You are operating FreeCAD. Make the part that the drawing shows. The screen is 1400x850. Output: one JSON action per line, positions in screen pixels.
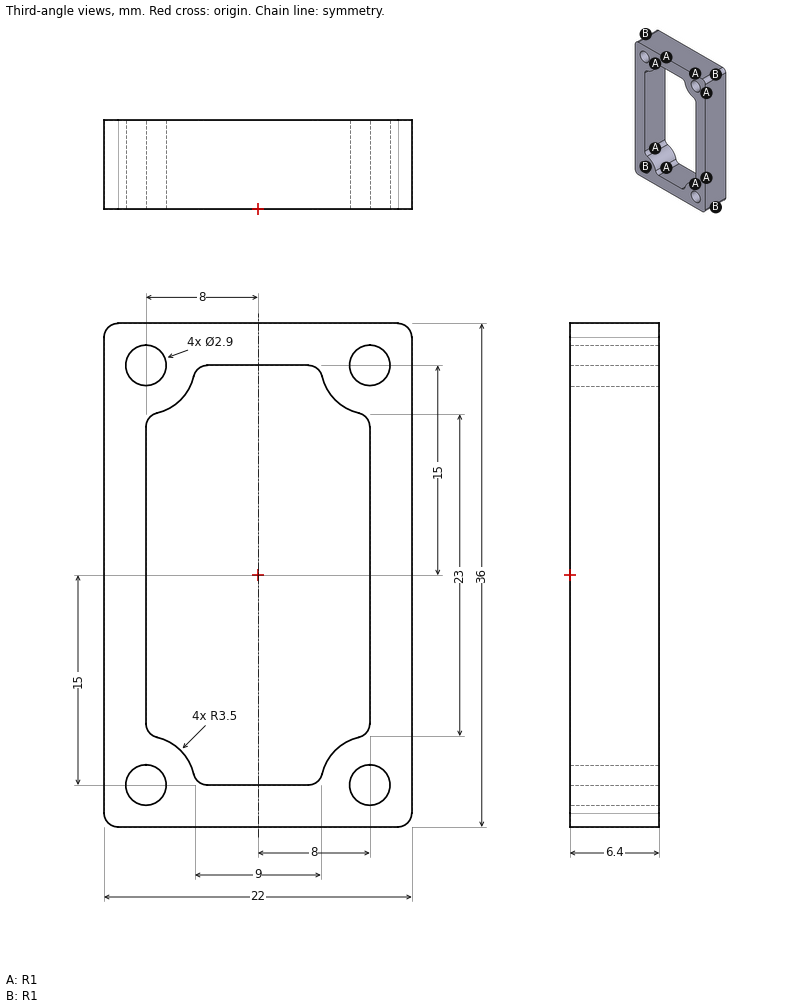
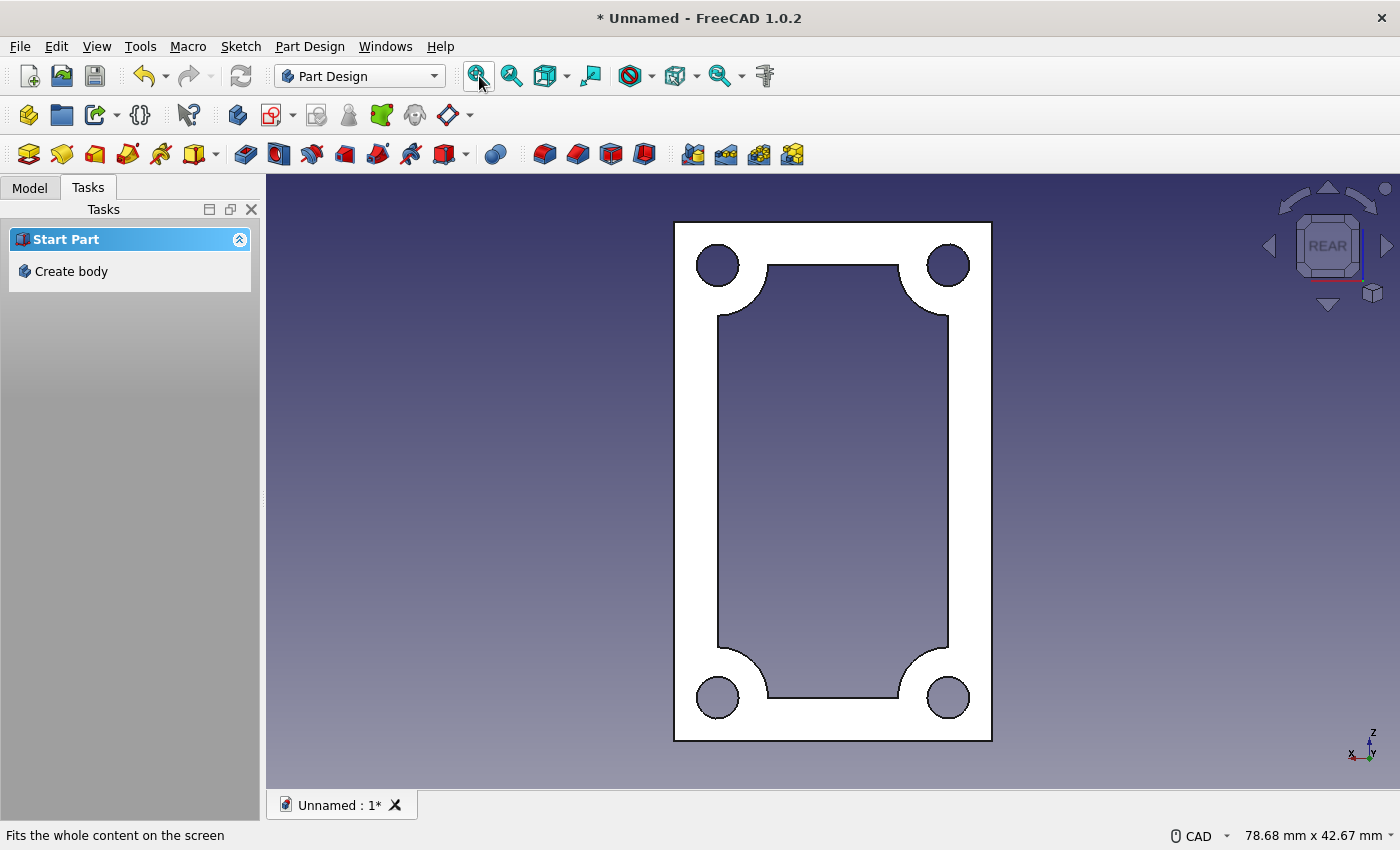
{"action": "key", "text": "6"}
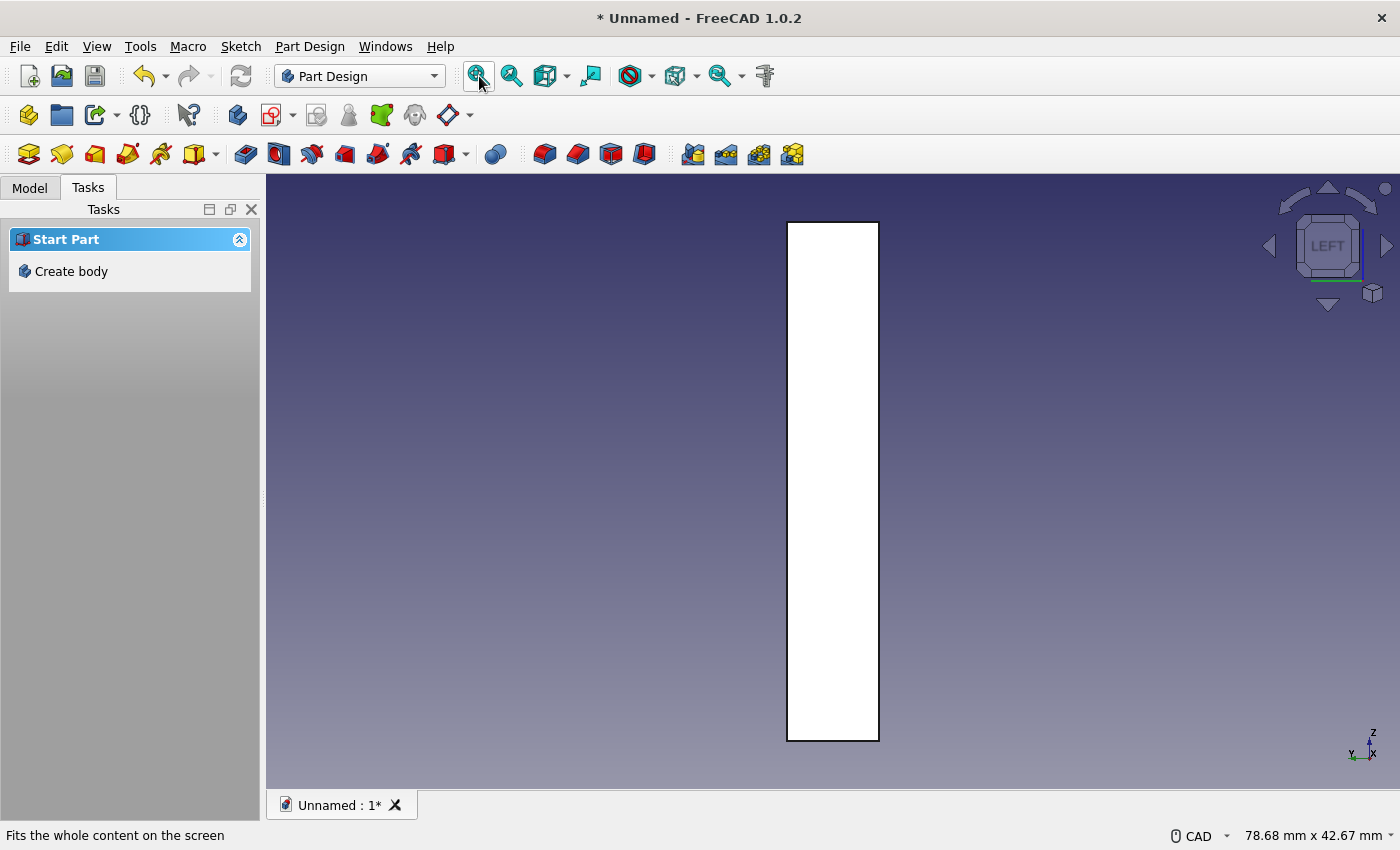
{"action": "key", "text": "v 3"}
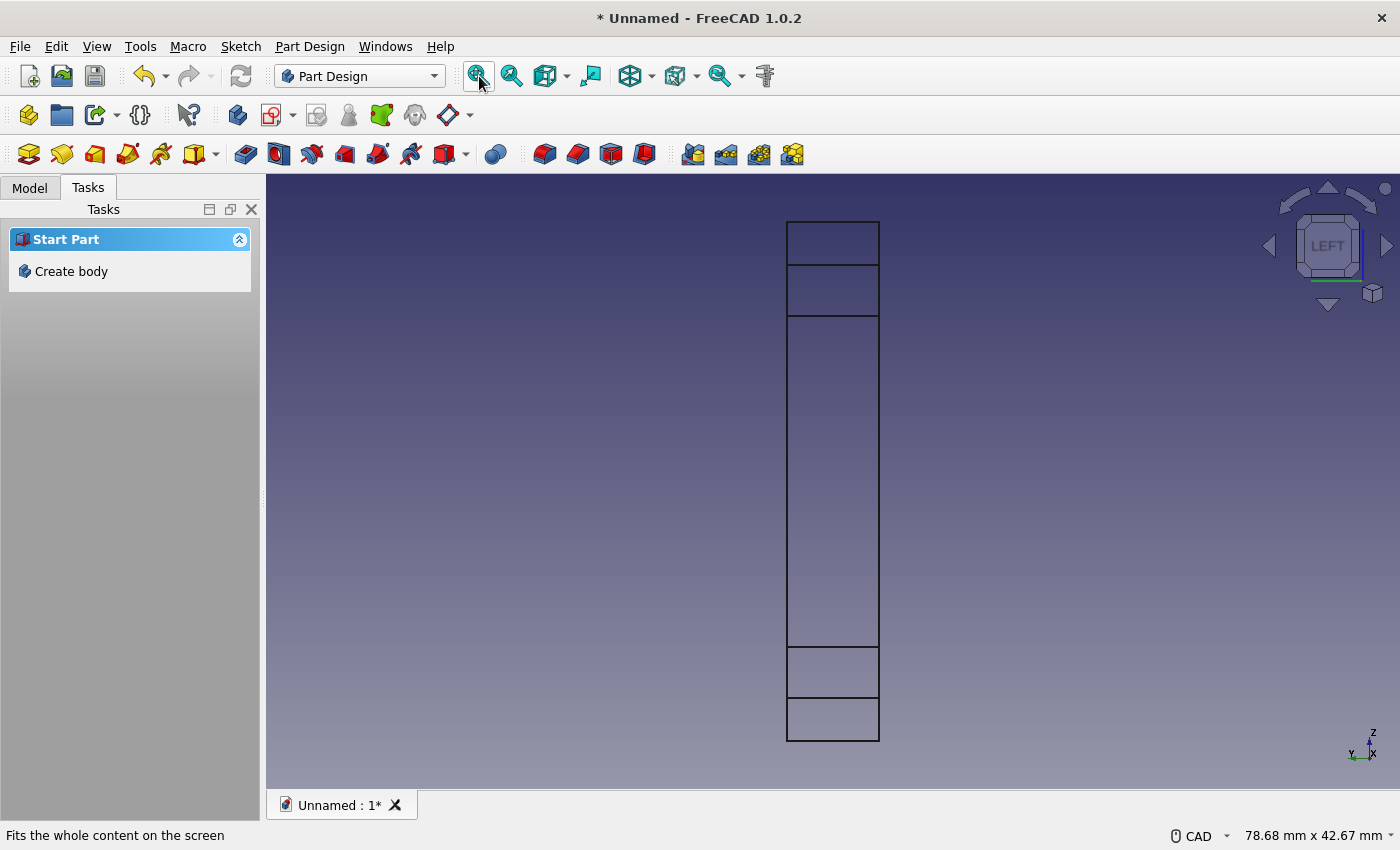
{"action": "key", "text": "0"}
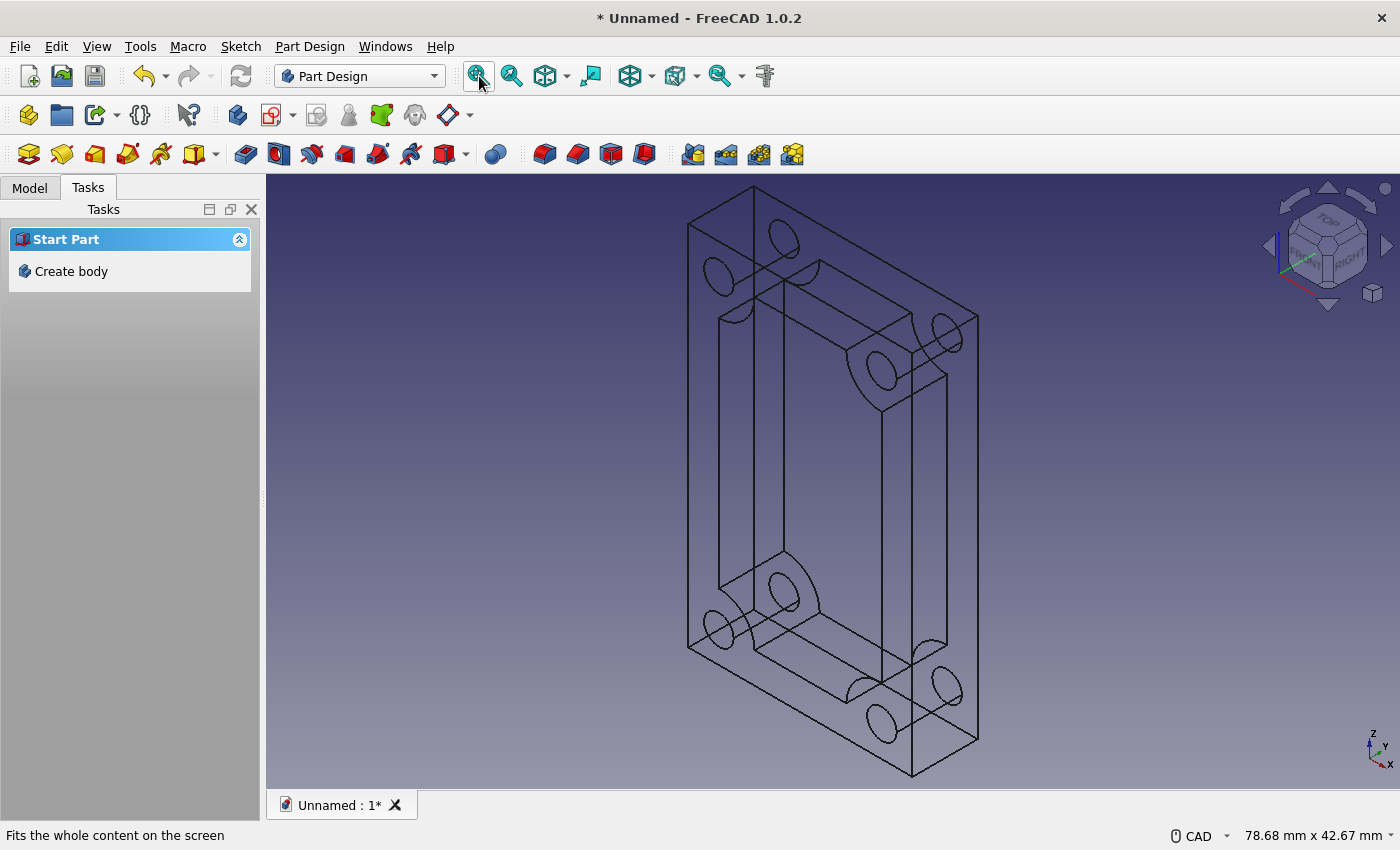
{"action": "left_click", "coordinate": [921, 659]}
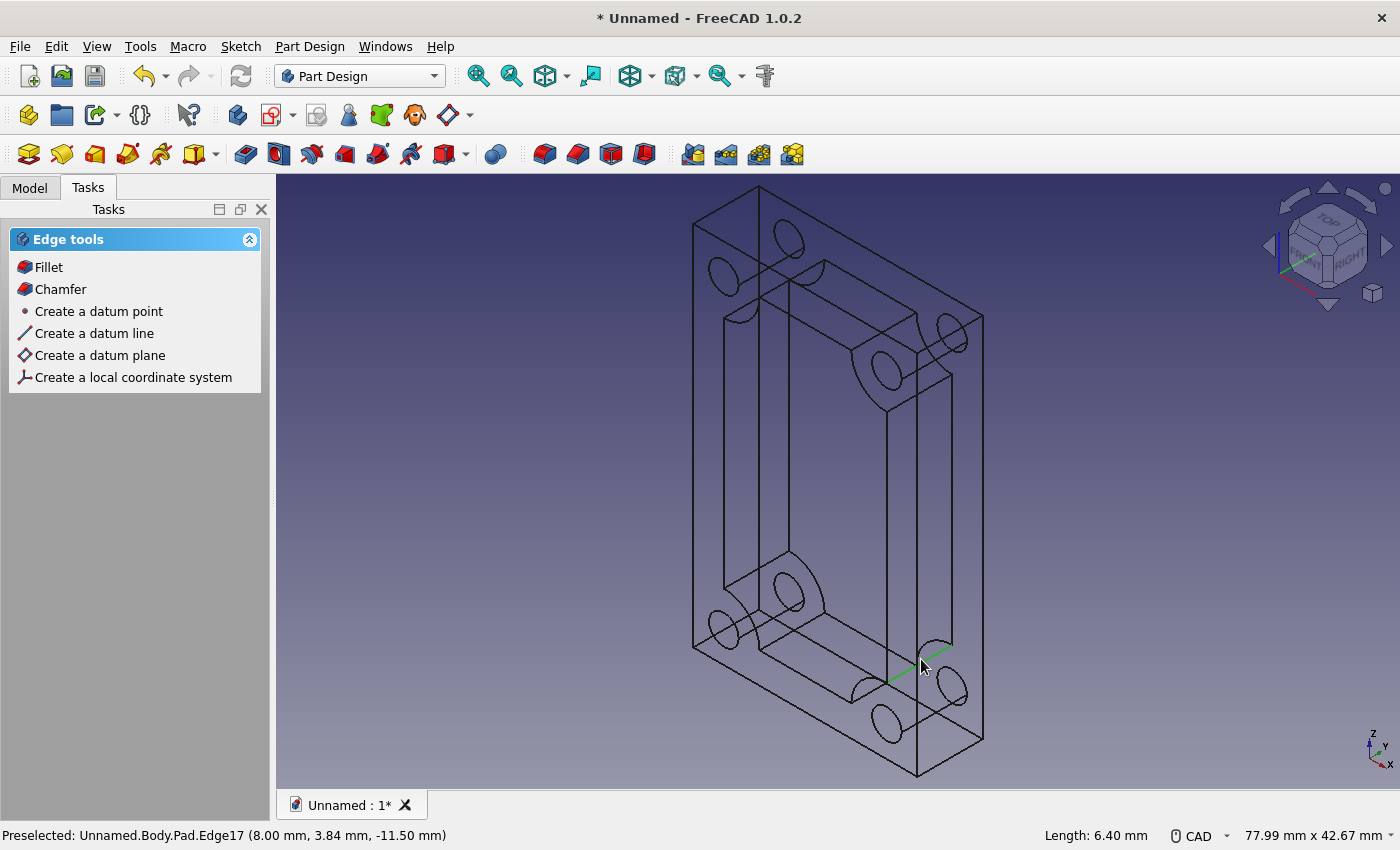
{"action": "left_click", "coordinate": [877, 687], "text": "ctrl"}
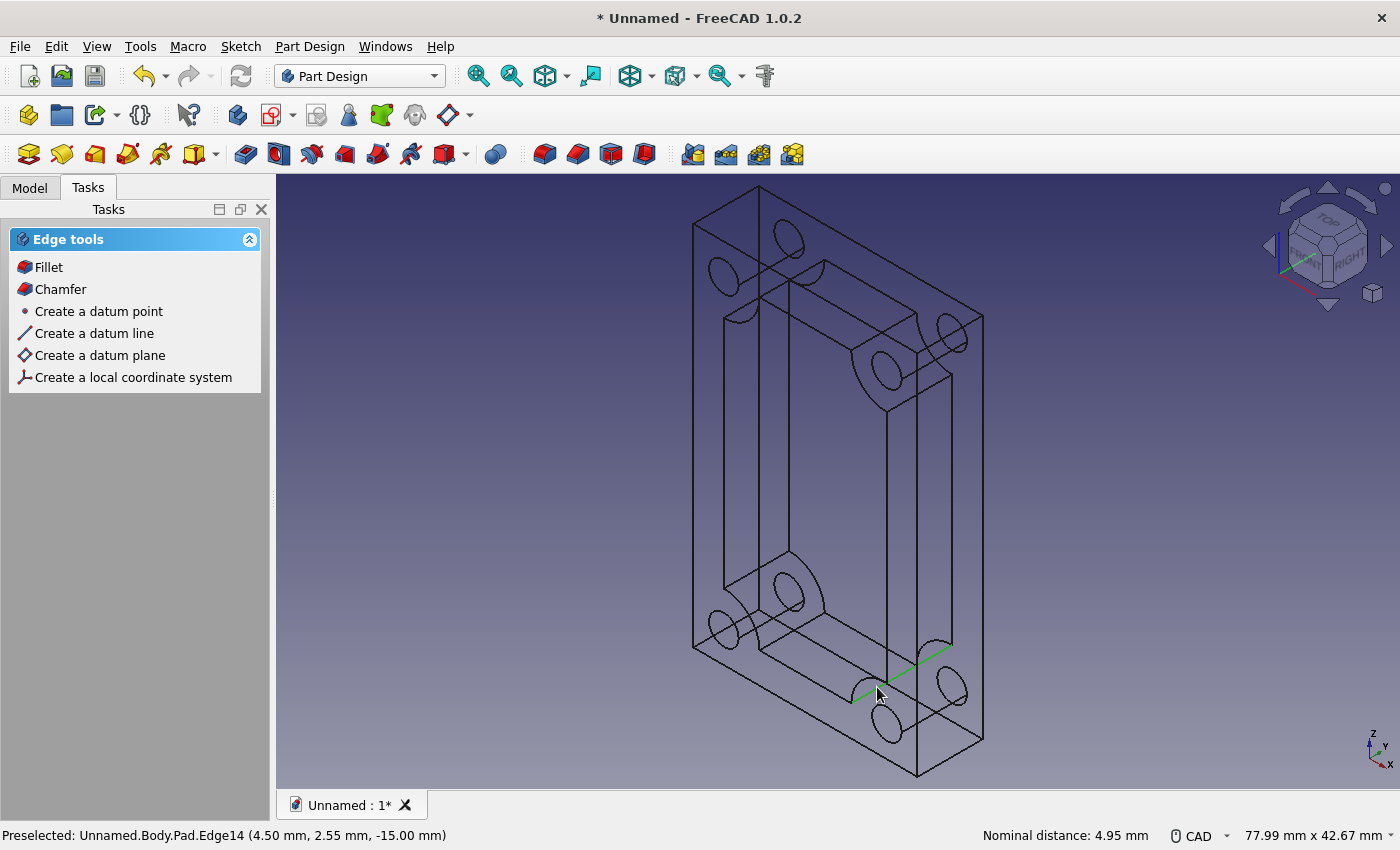
{"action": "left_click", "coordinate": [792, 631], "text": "ctrl"}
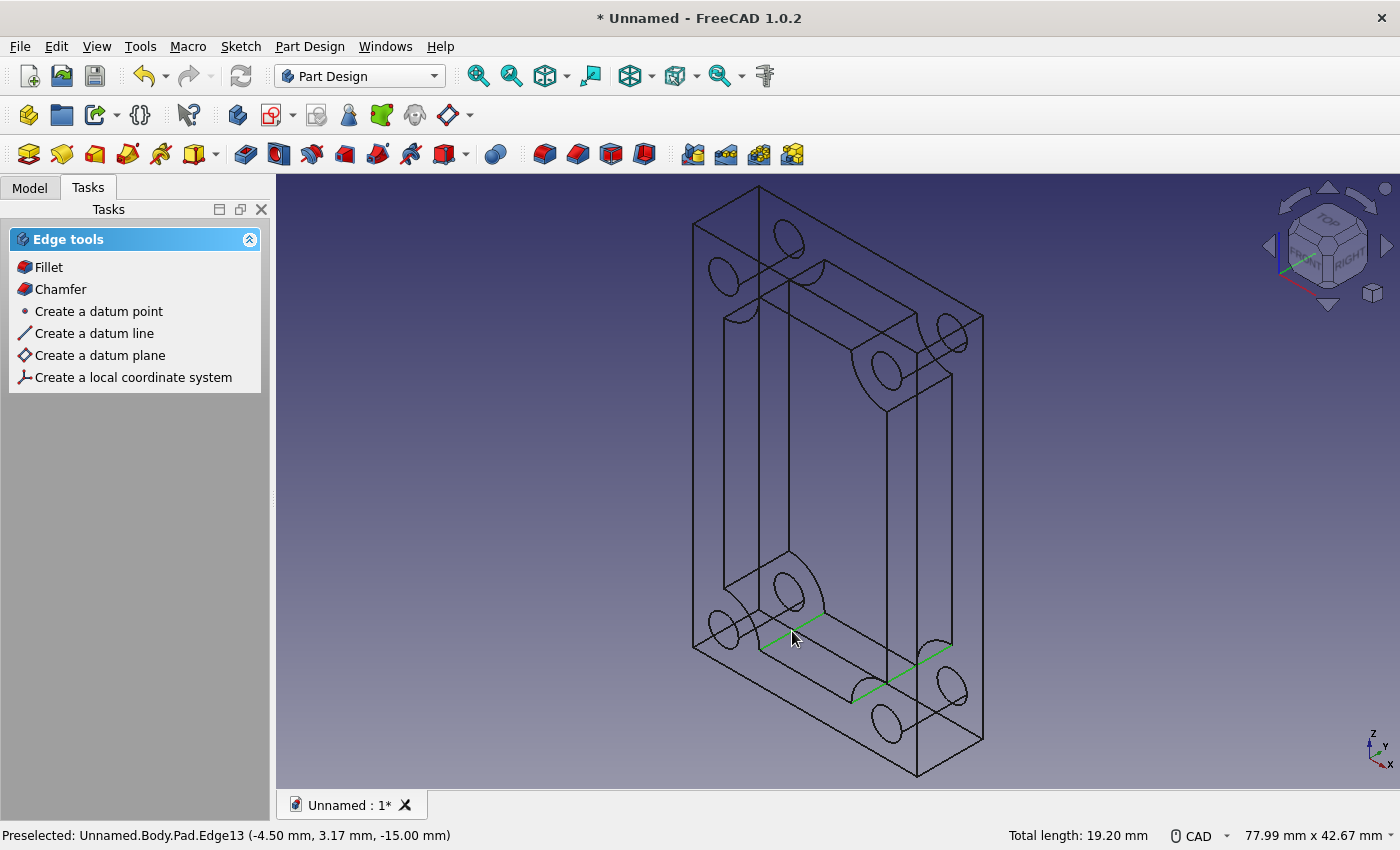
{"action": "left_click", "coordinate": [756, 569], "text": "ctrl"}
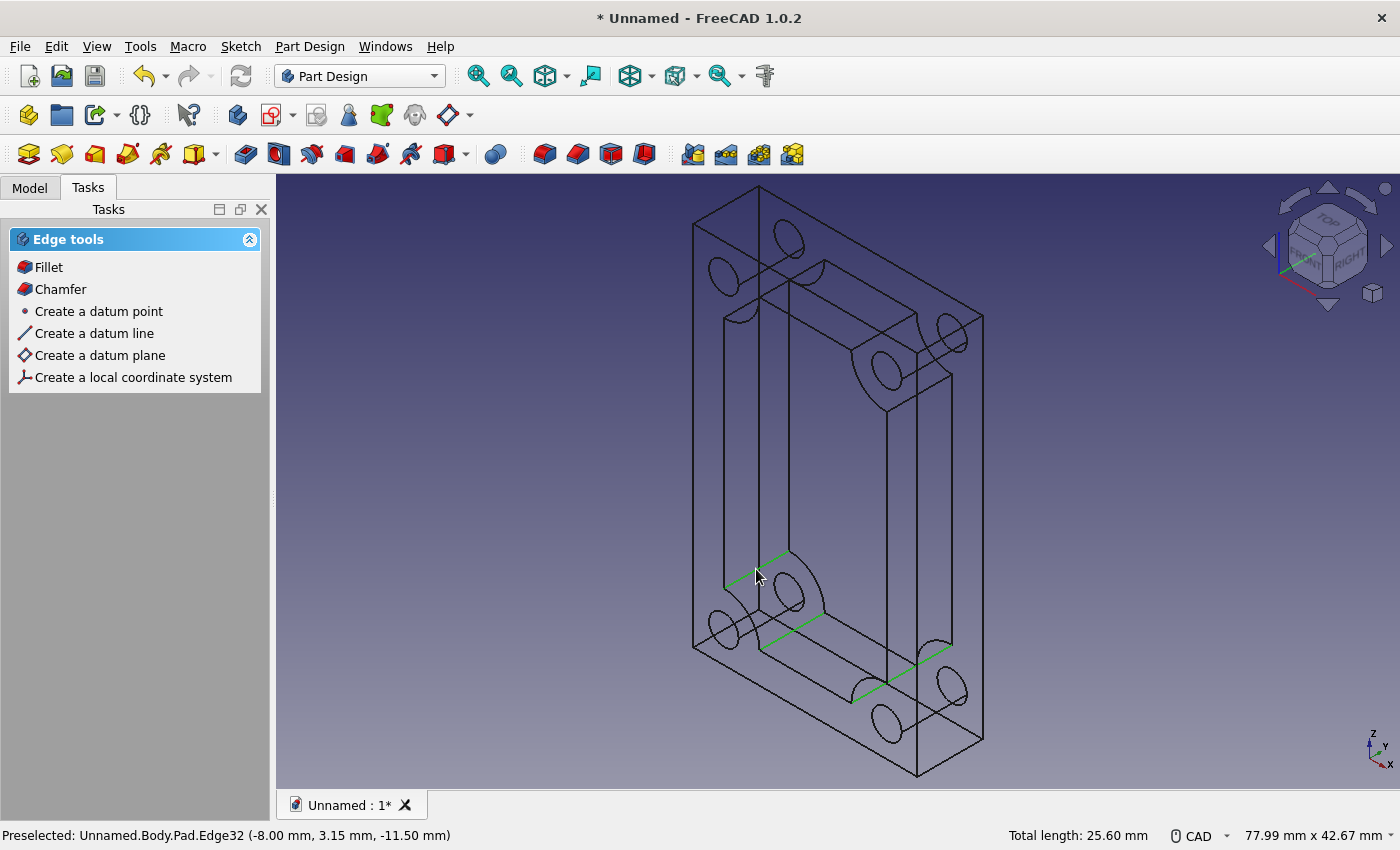
{"action": "left_click", "coordinate": [750, 302], "text": "ctrl"}